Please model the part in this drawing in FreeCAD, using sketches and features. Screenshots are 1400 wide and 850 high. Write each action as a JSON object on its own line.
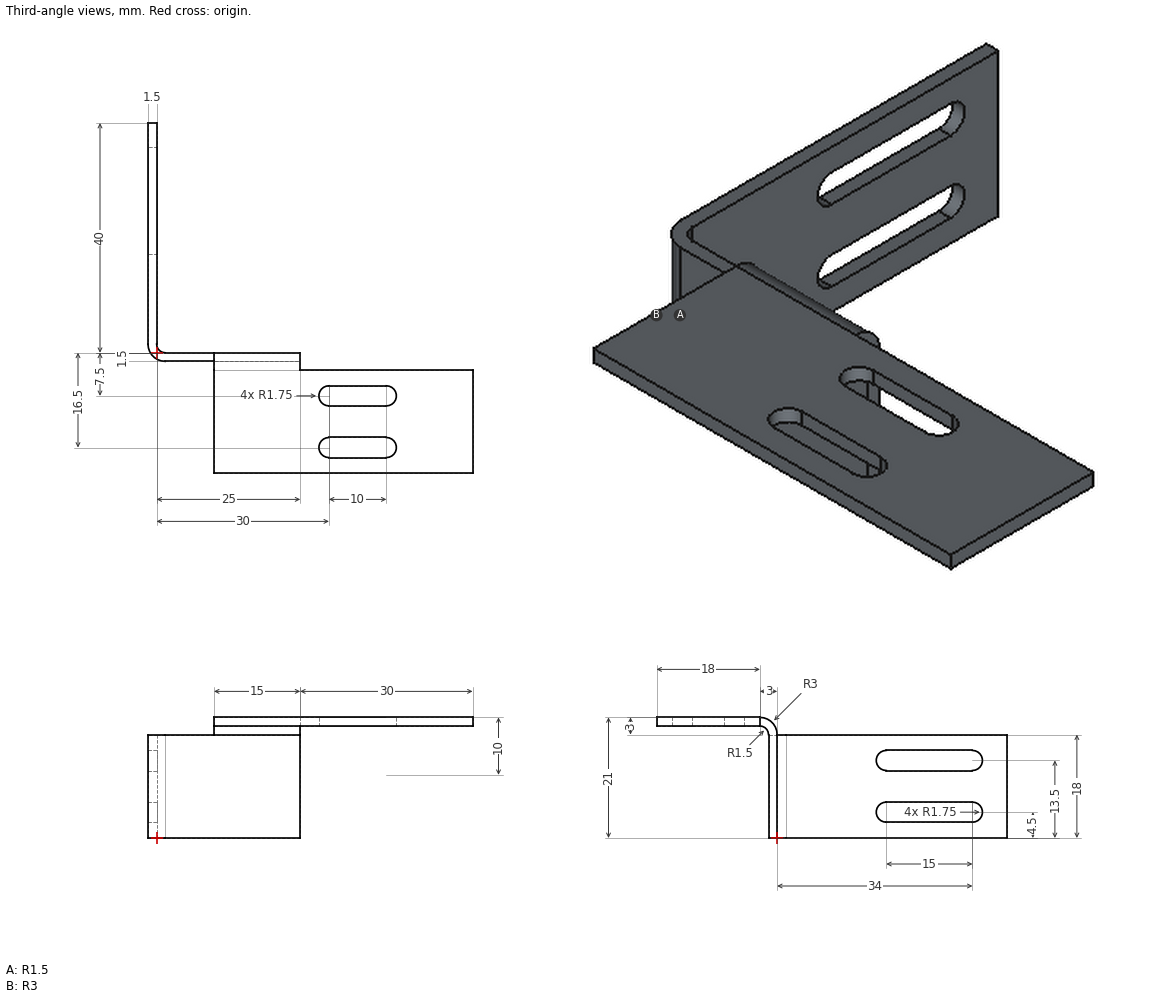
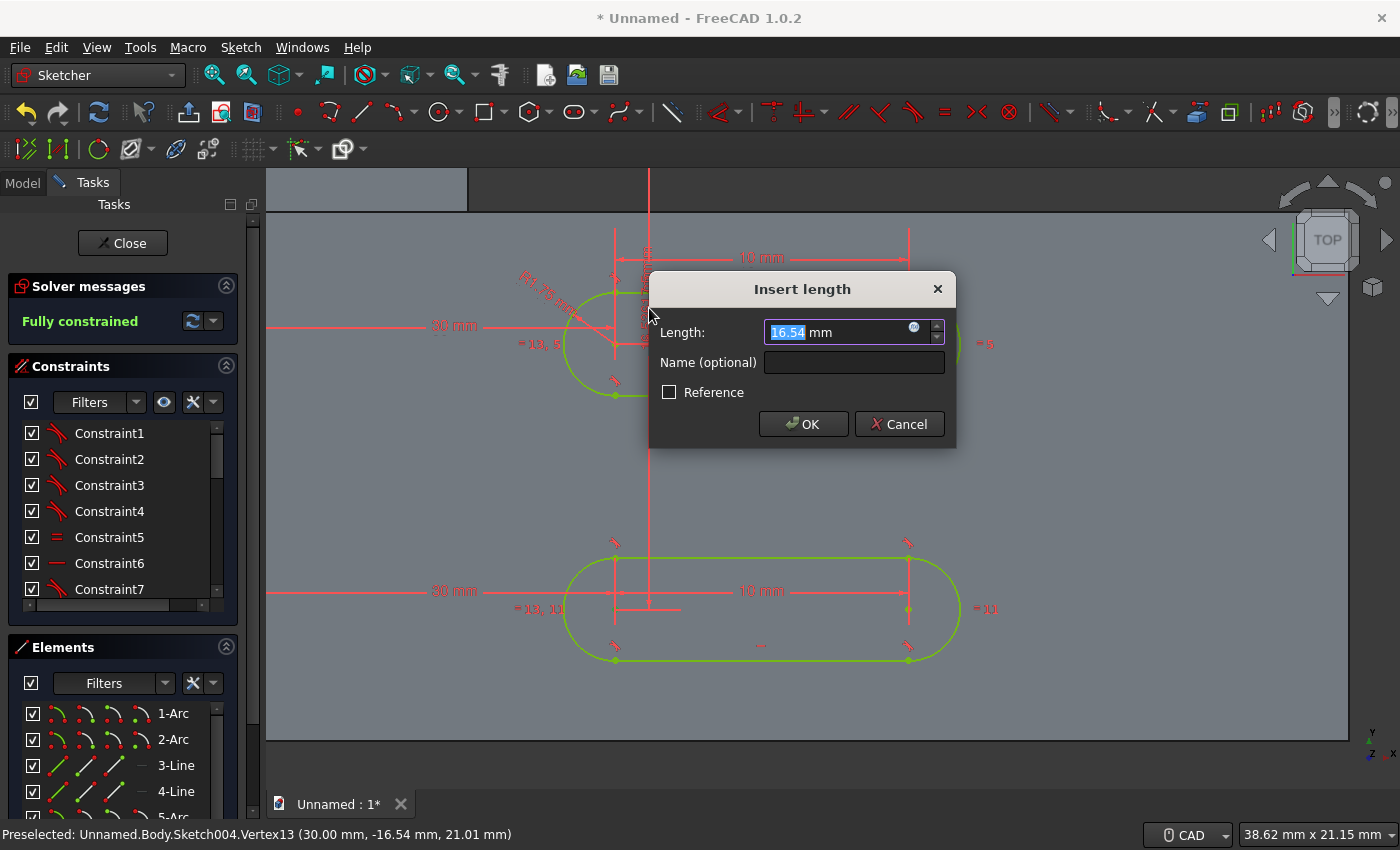
{"action": "type", "text": "16.5"}
{"action": "key", "text": "Return"}
{"action": "key", "text": "Escape"}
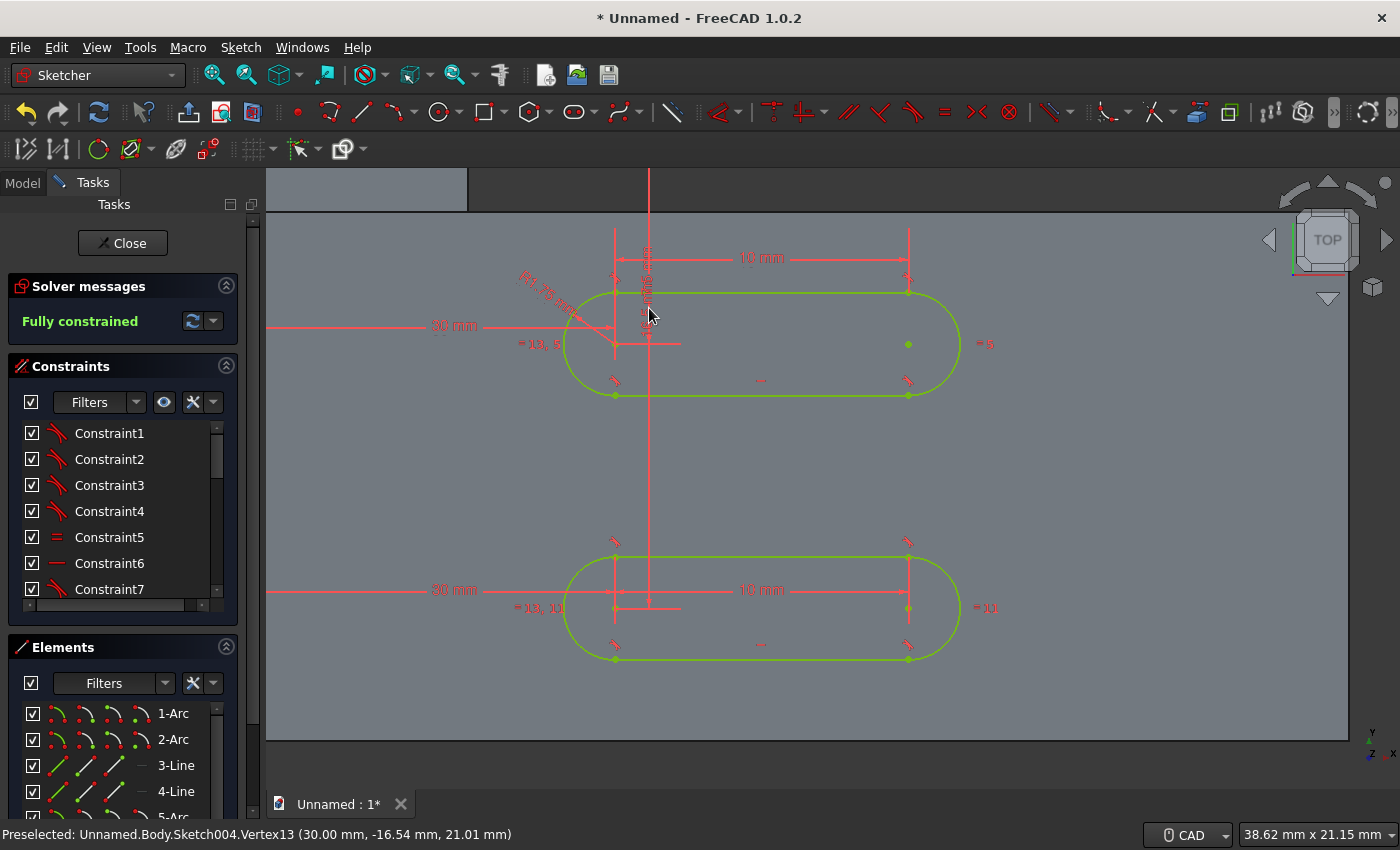
{"action": "left_click", "coordinate": [123, 243]}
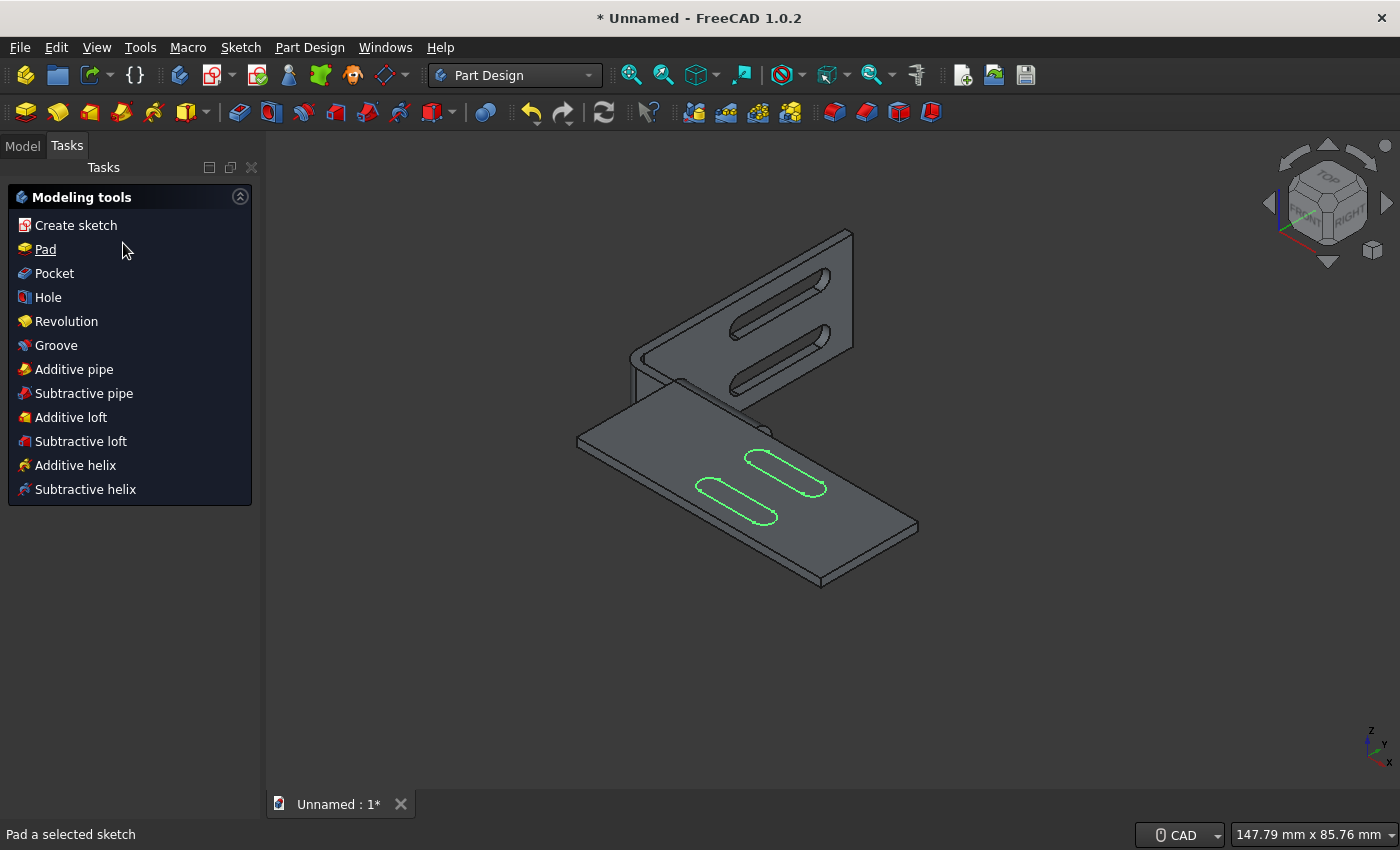
{"action": "left_click", "coordinate": [240, 112]}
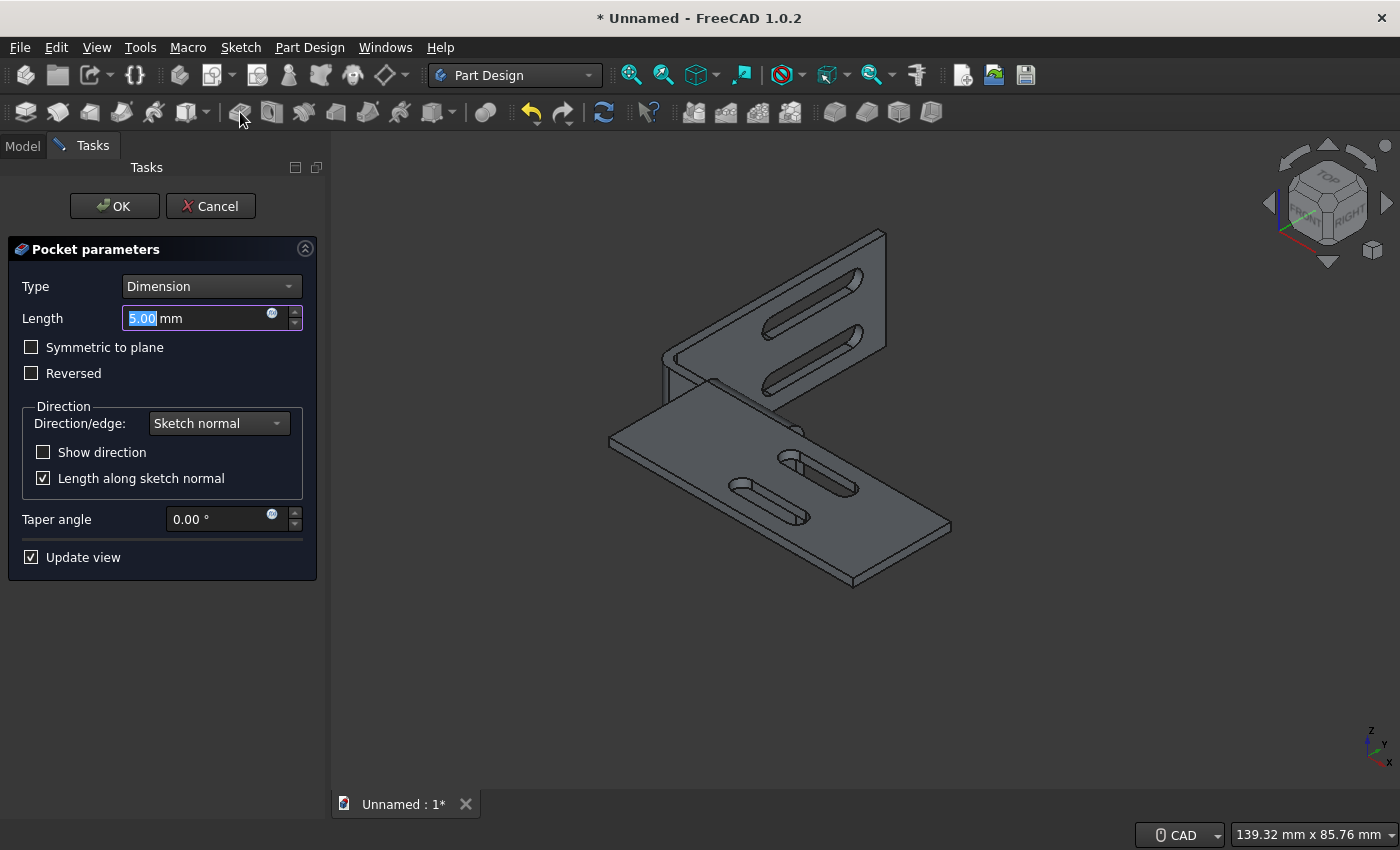
{"action": "type", "text": "10"}
{"action": "key", "text": "Tab"}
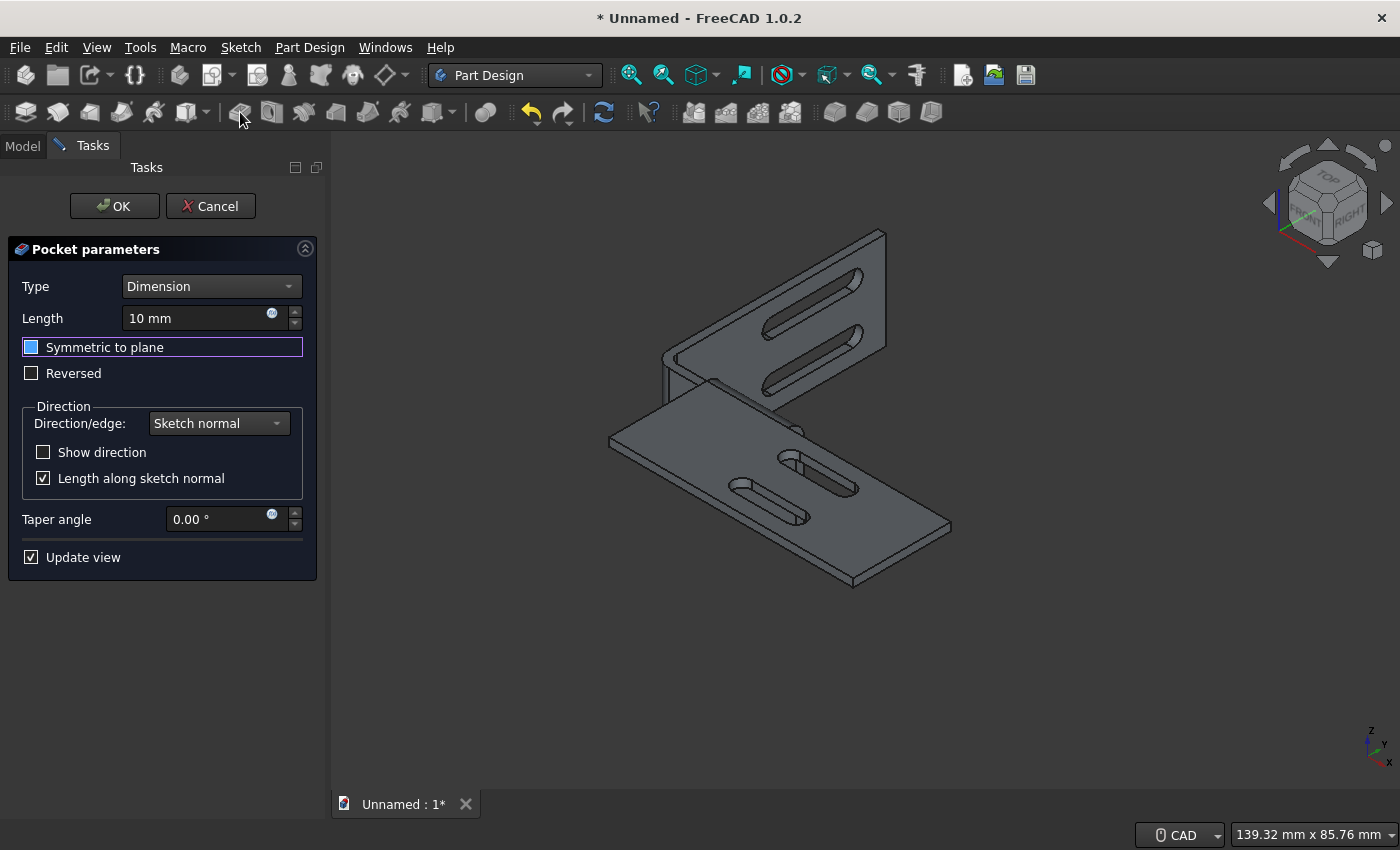
{"action": "left_click", "coordinate": [115, 206]}